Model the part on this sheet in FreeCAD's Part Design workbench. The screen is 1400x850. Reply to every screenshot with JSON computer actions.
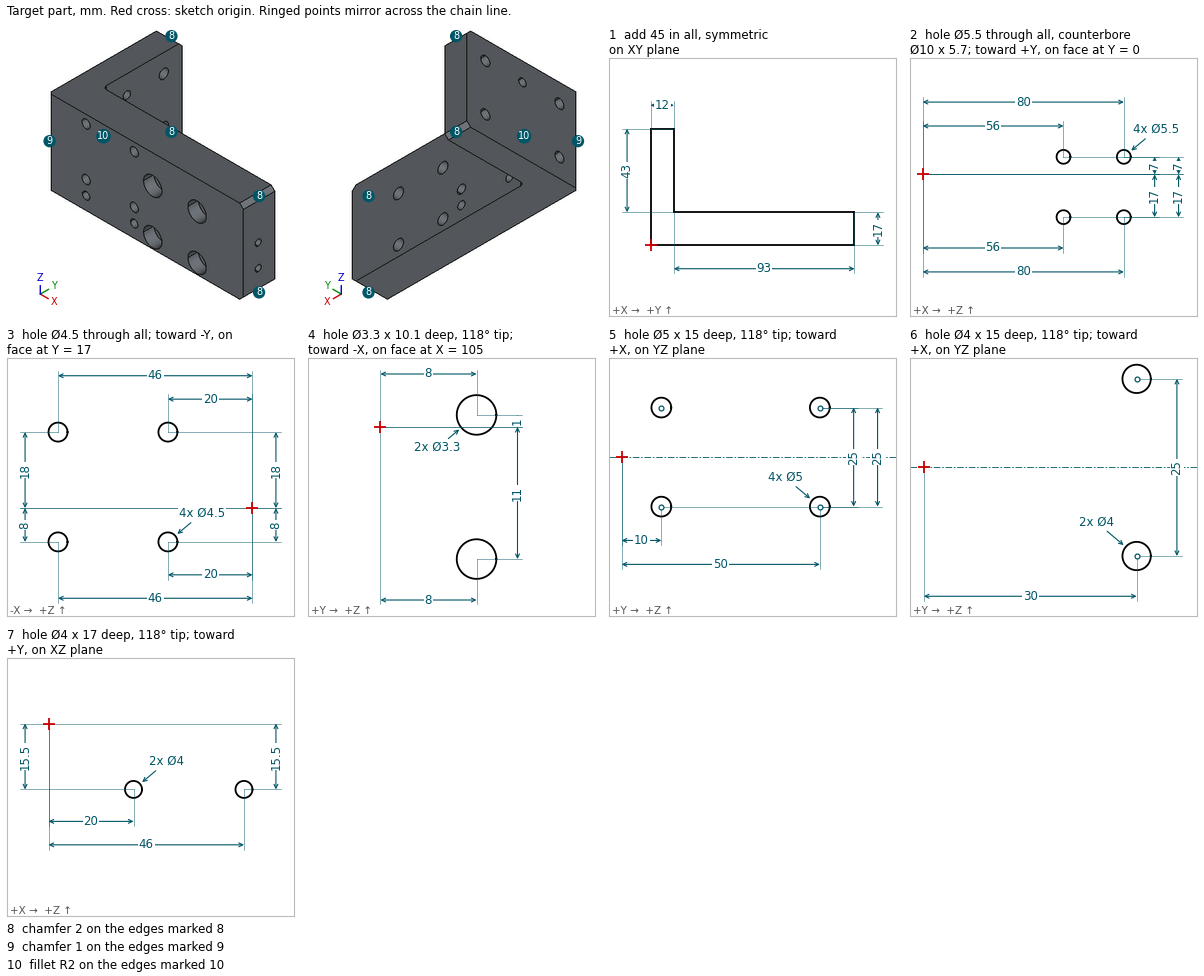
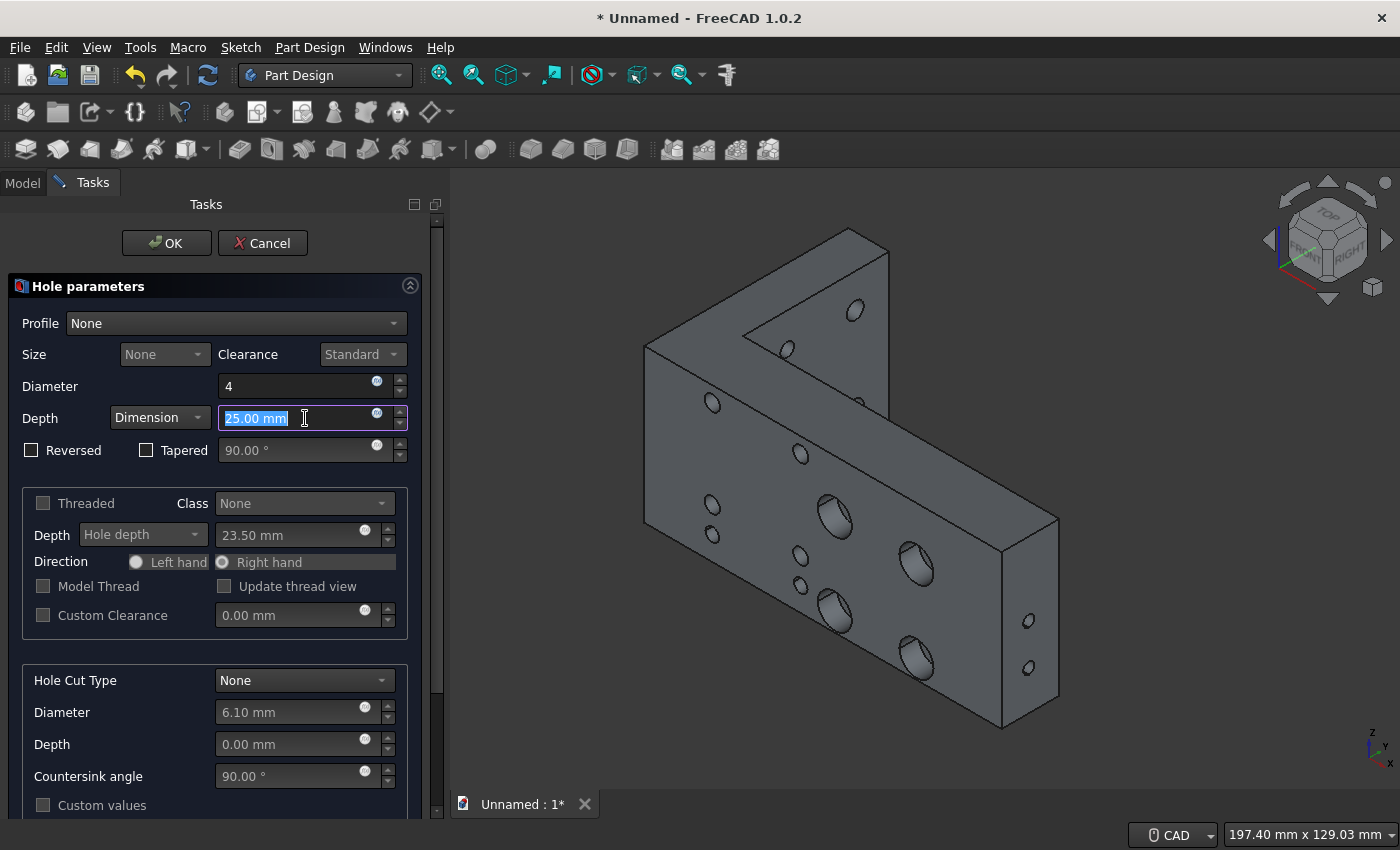
{"action": "type", "text": "17"}
{"action": "key", "text": "Tab"}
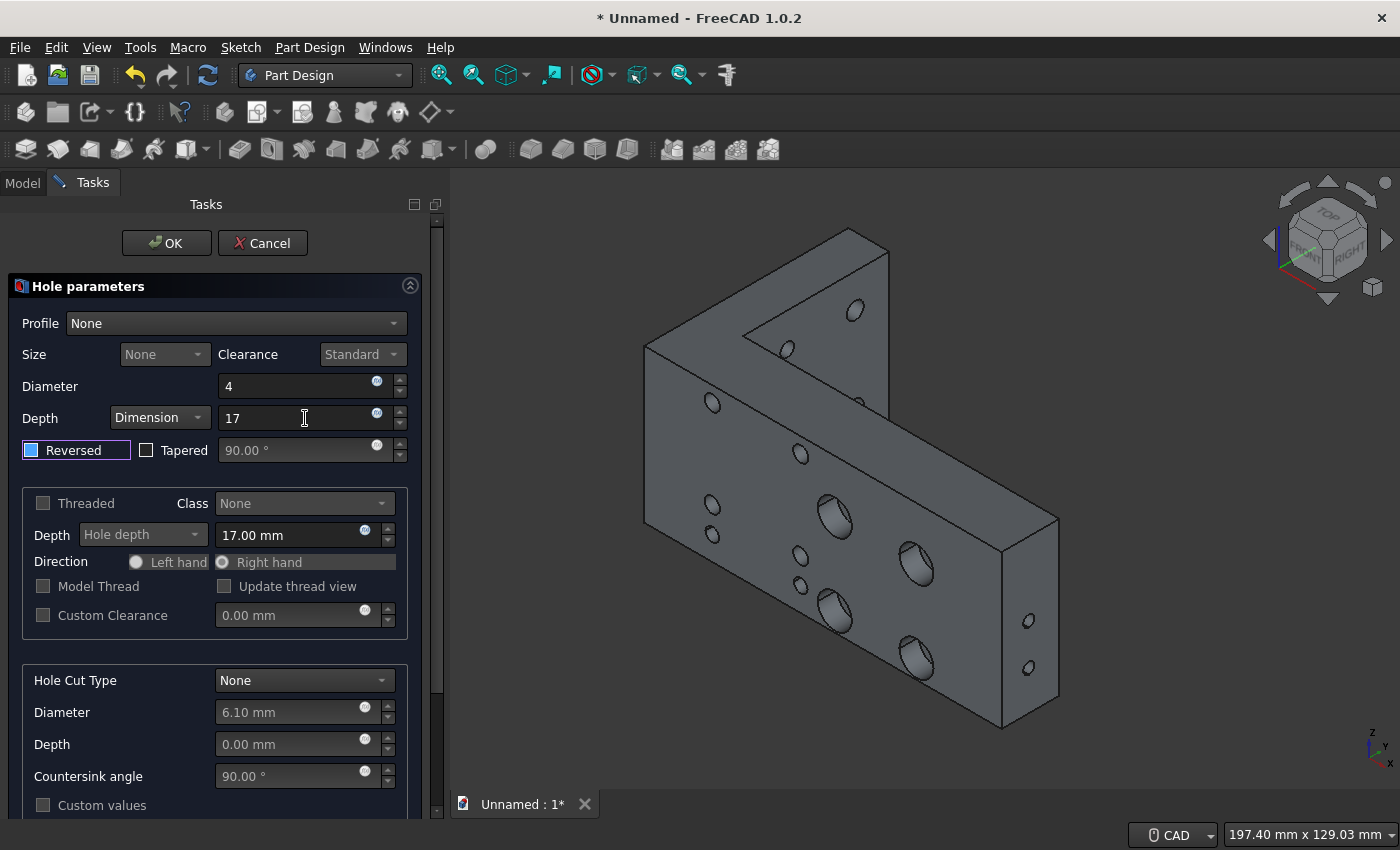
{"action": "left_click", "coordinate": [167, 243]}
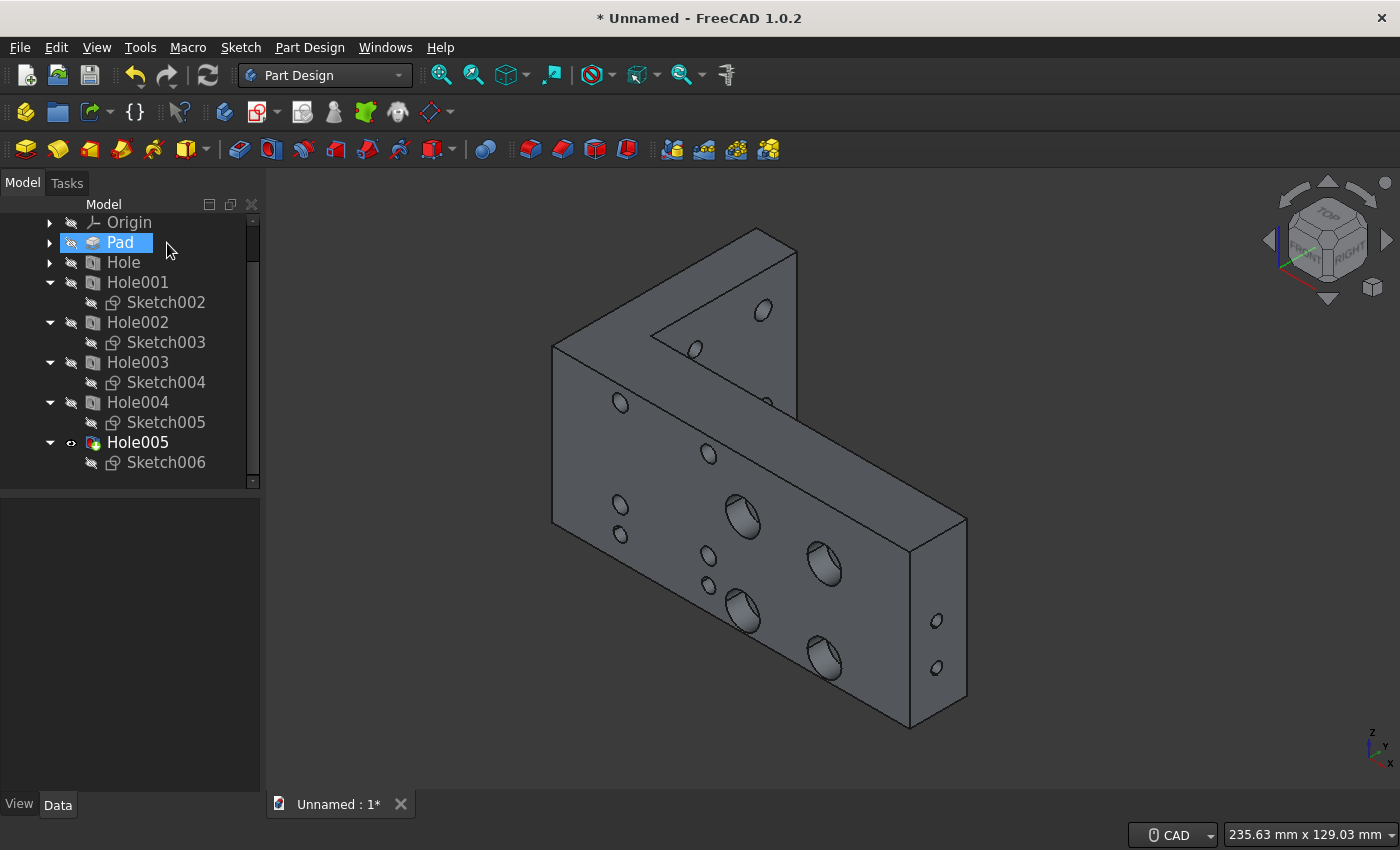
{"action": "left_click", "coordinate": [938, 534]}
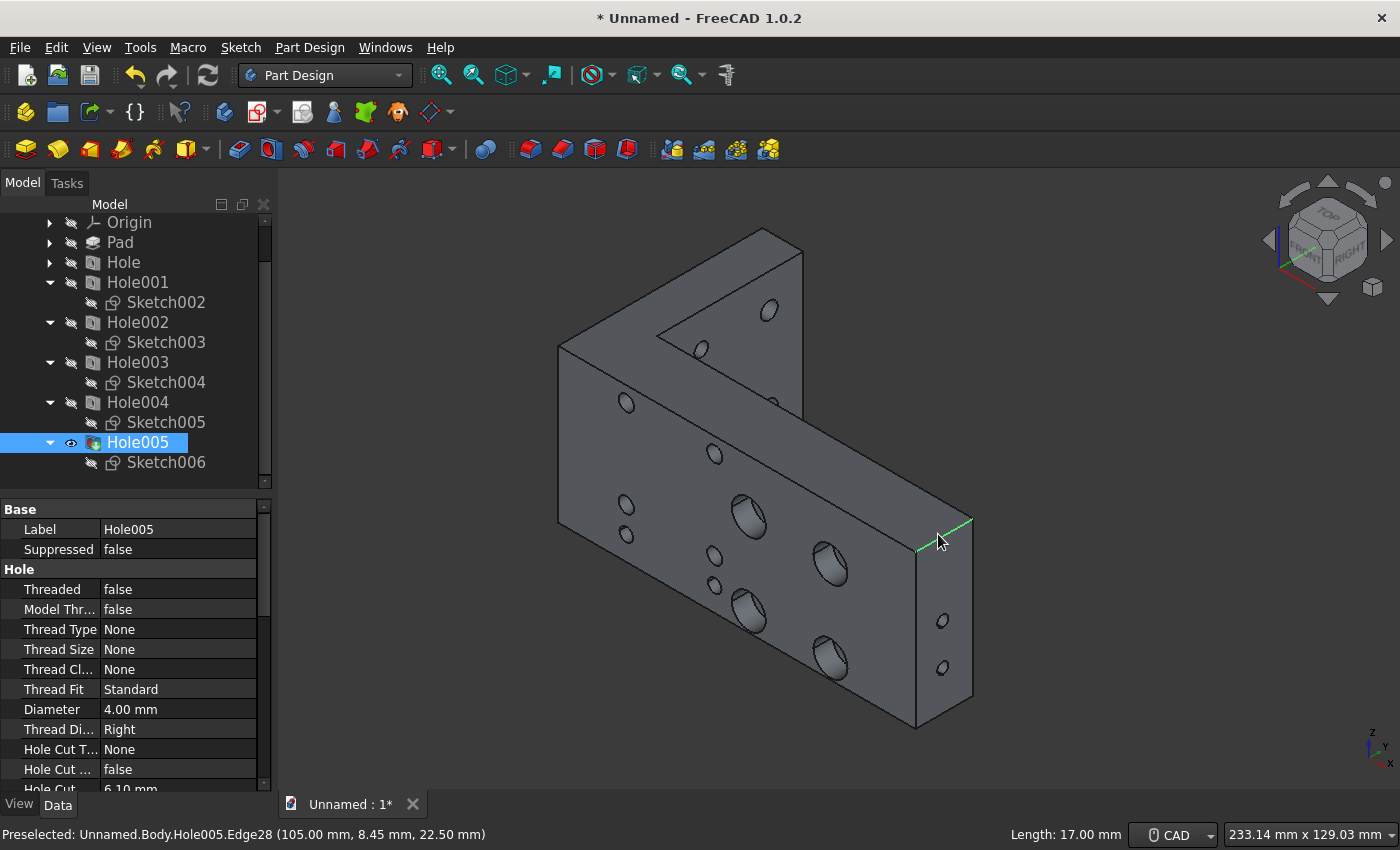
{"action": "key", "text": "2"}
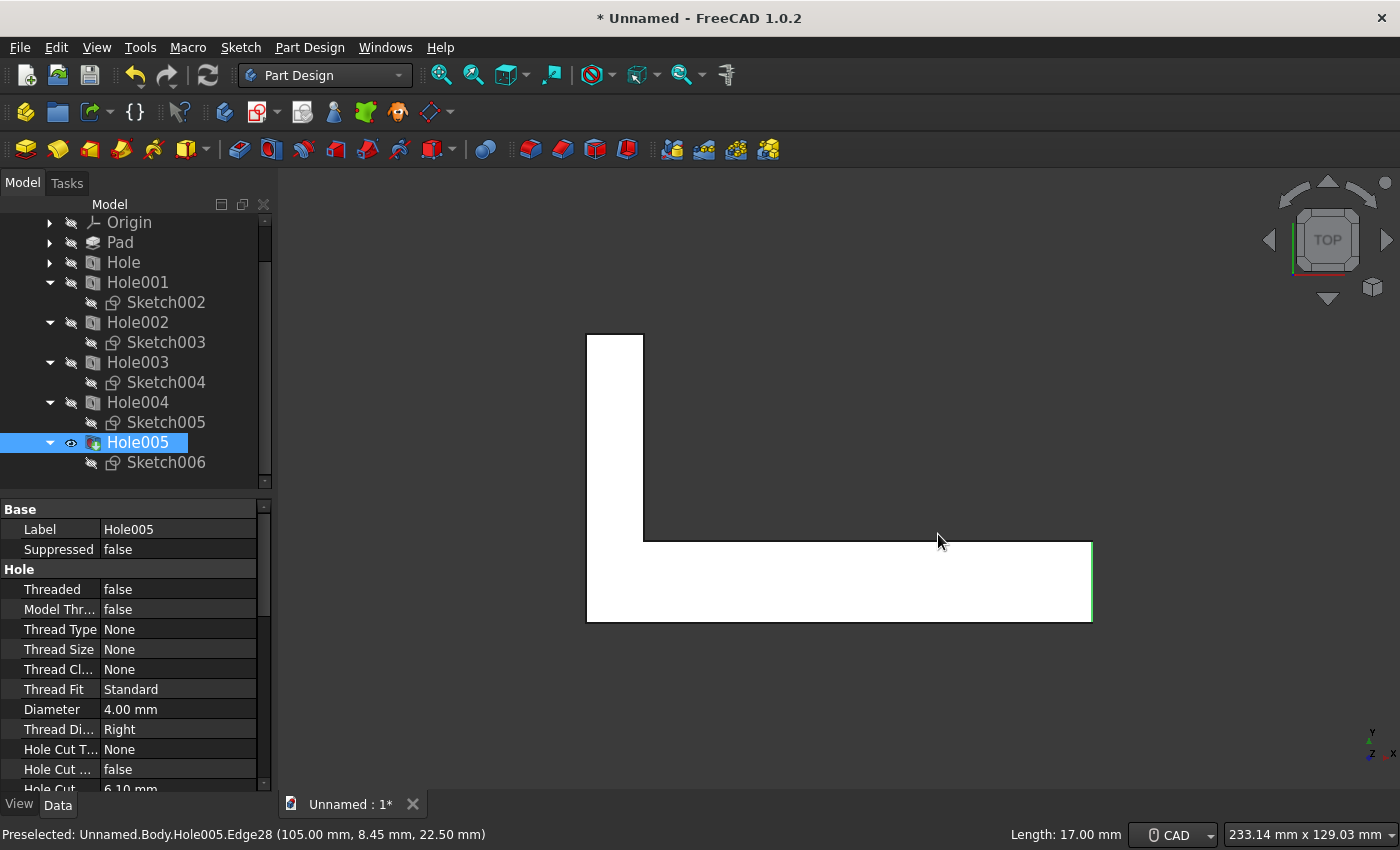
{"action": "left_click", "coordinate": [615, 333], "text": "ctrl"}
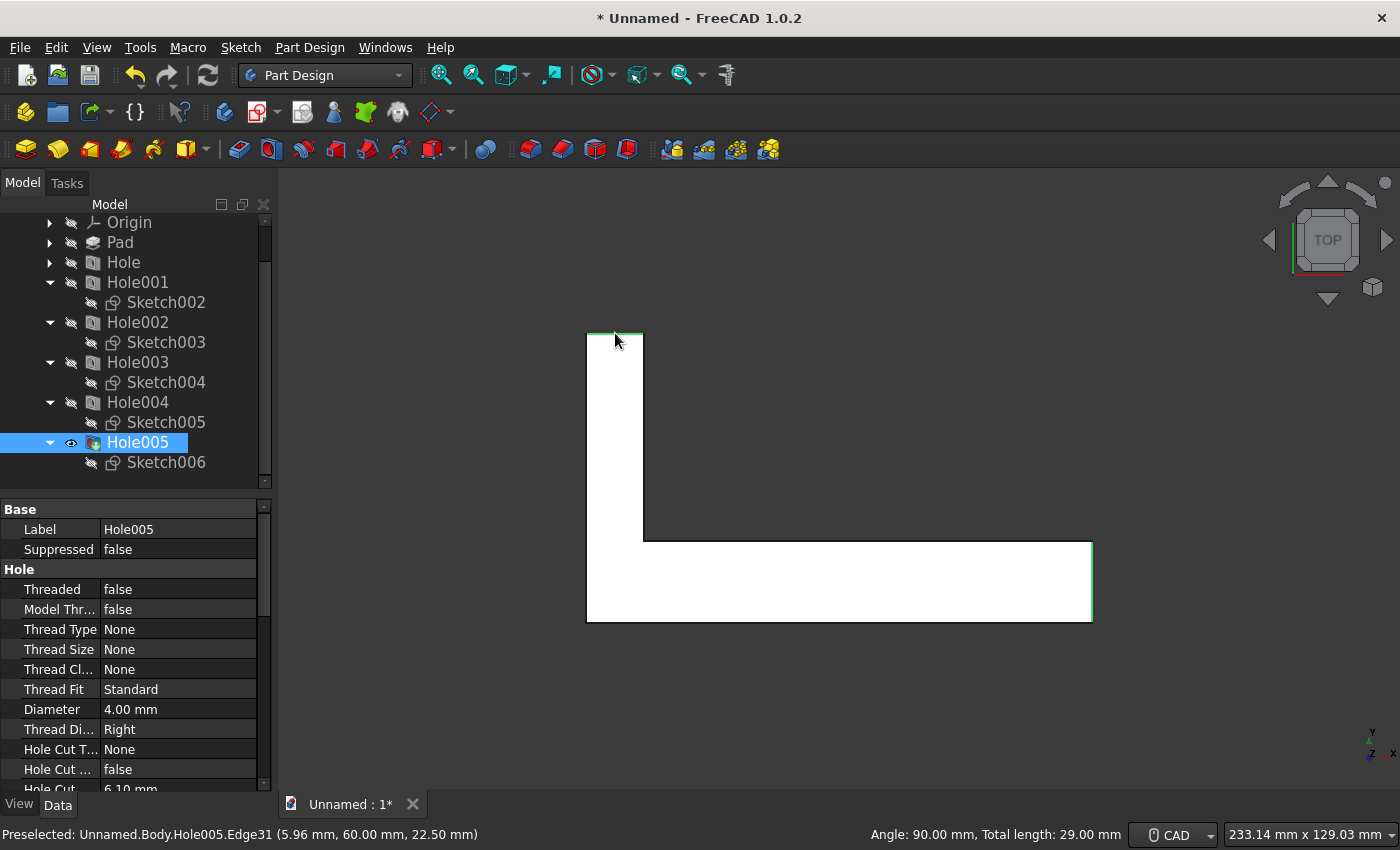
{"action": "key", "text": "0"}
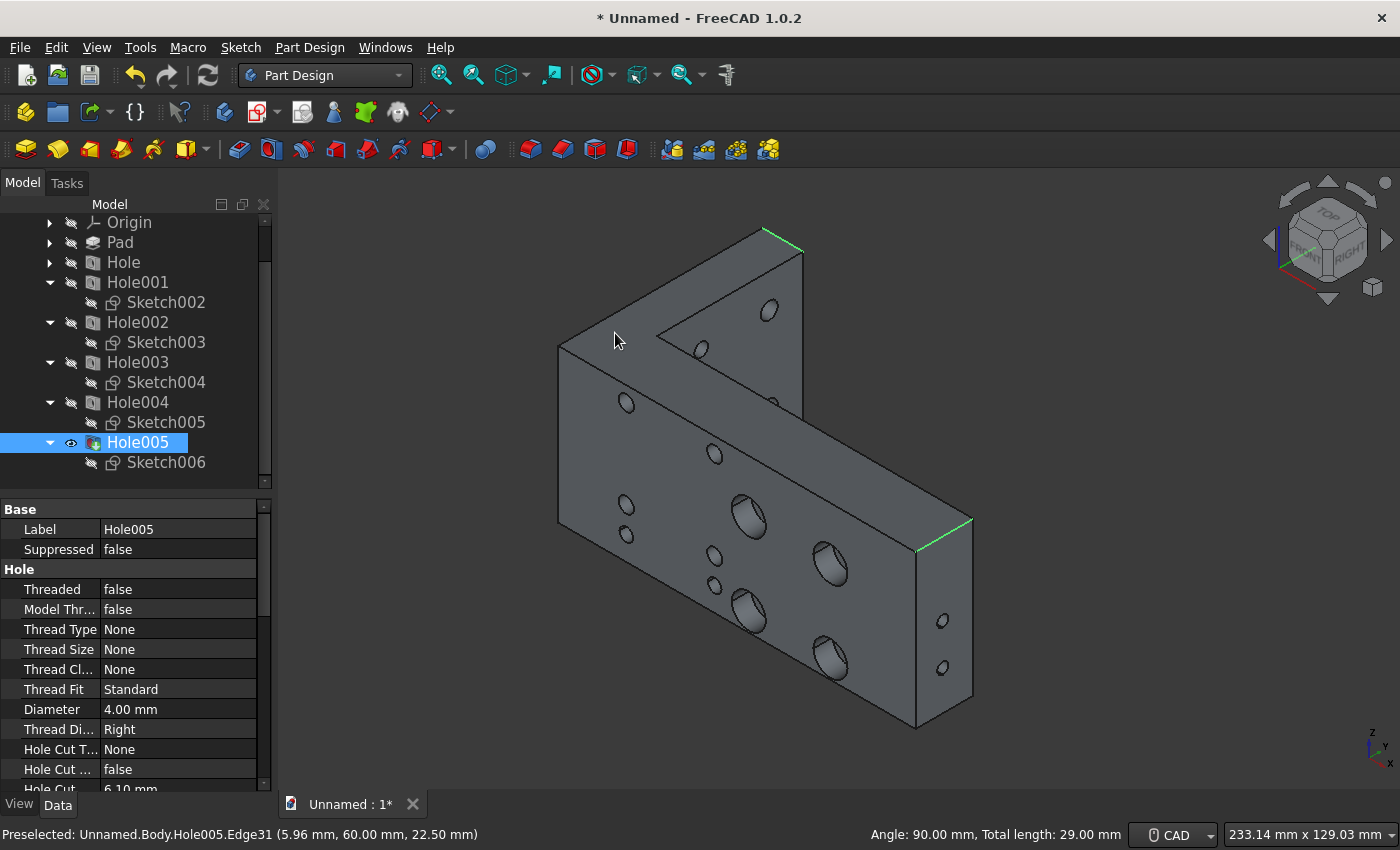
{"action": "key", "text": "1"}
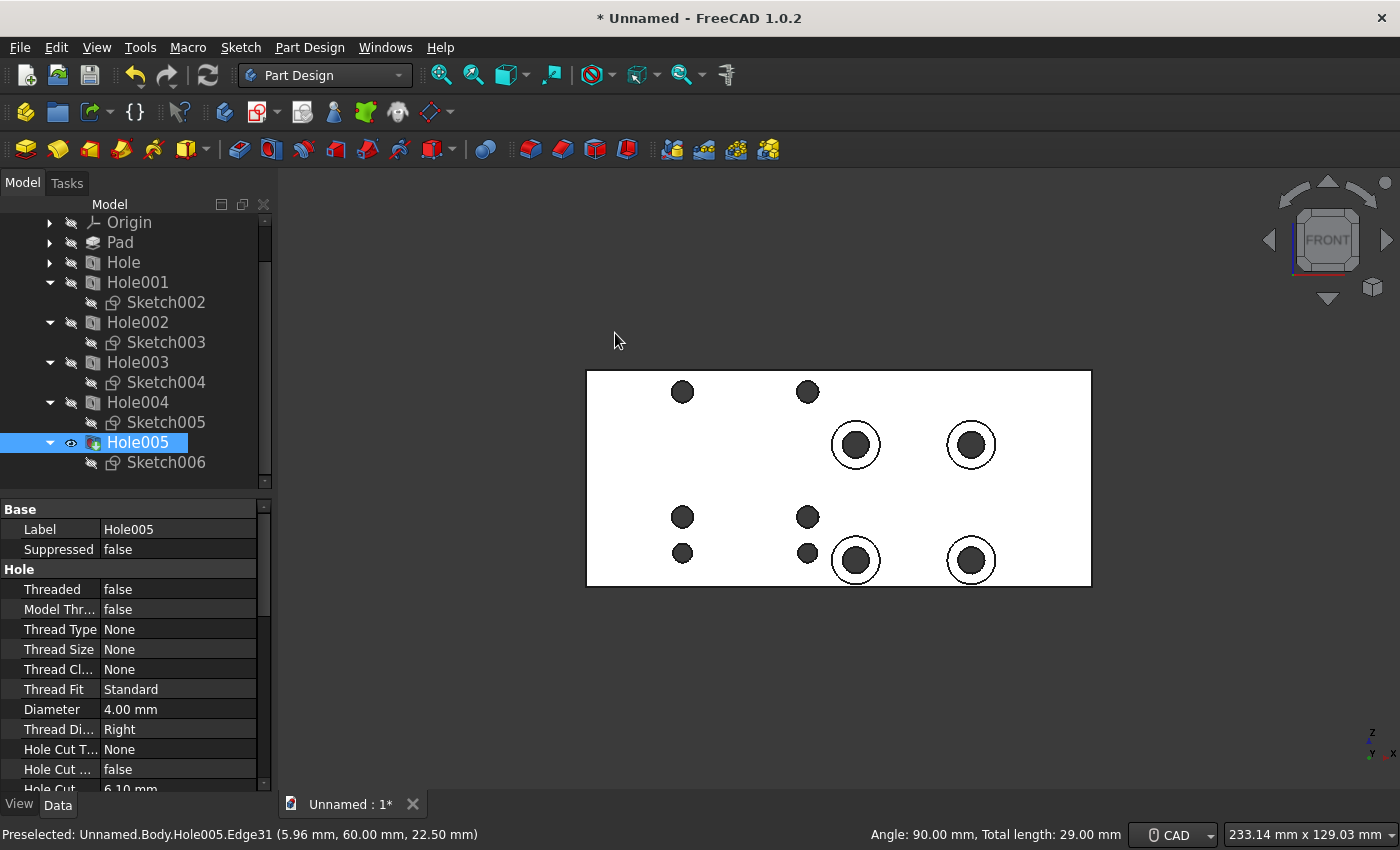
{"action": "key", "text": "3"}